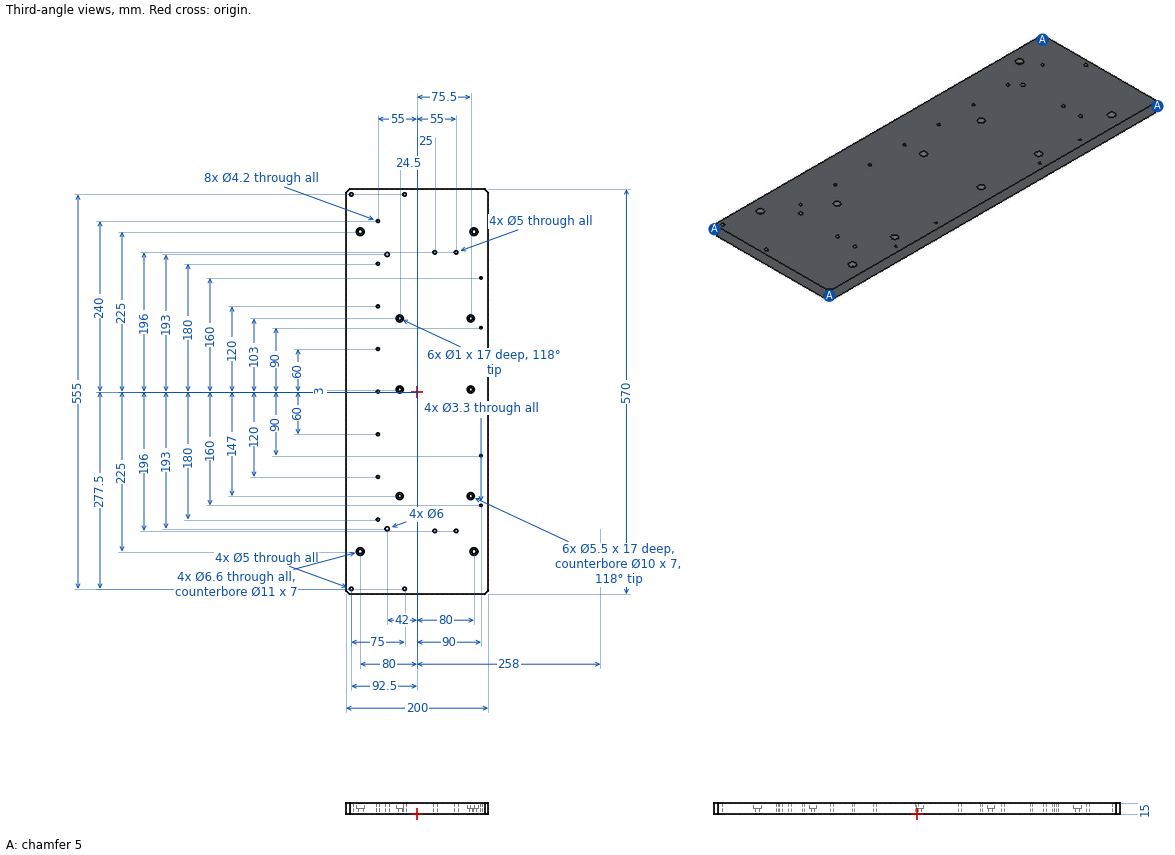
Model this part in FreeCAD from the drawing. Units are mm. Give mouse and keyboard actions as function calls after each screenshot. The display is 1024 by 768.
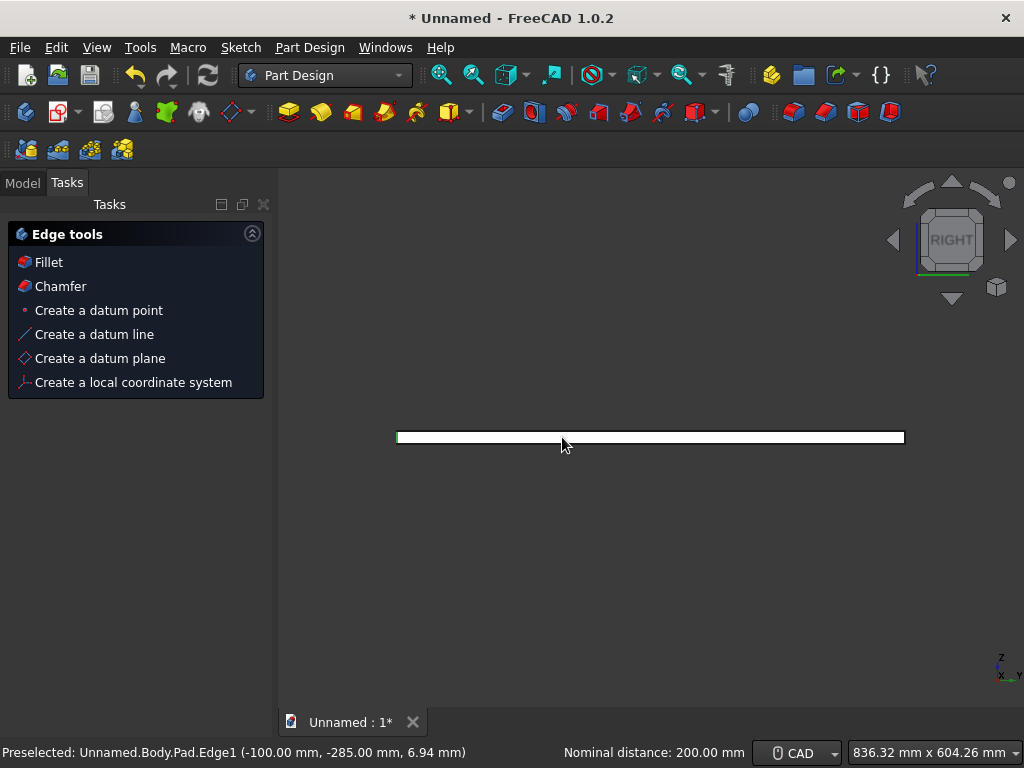
click(905, 436, ctrl)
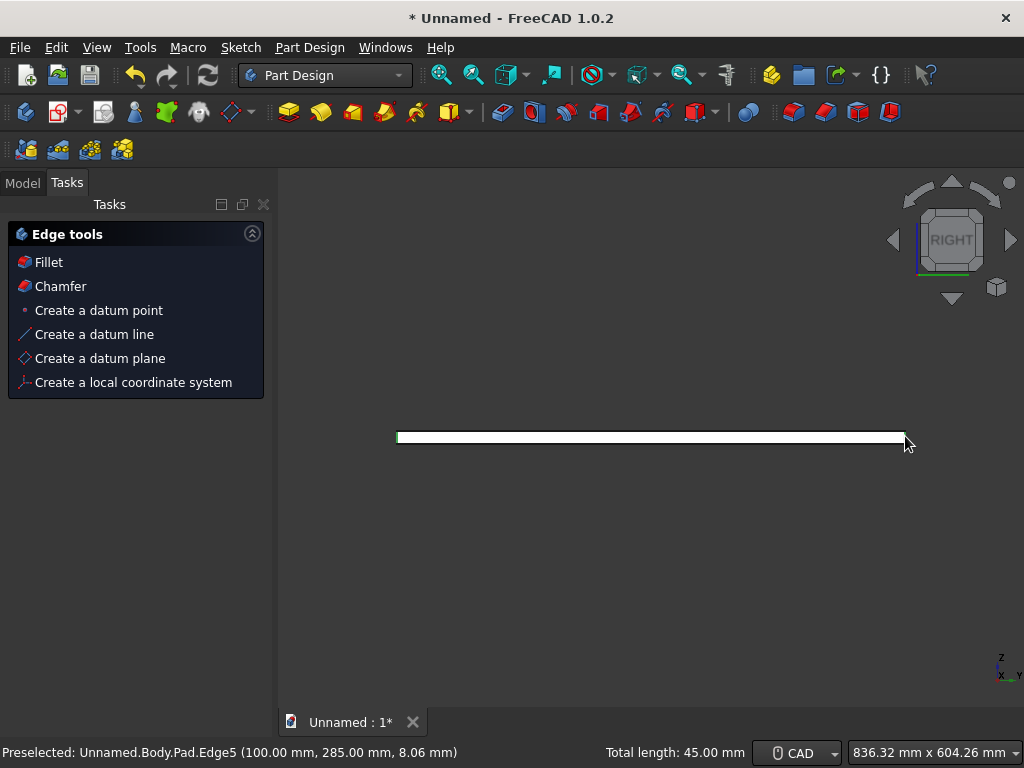
key(5)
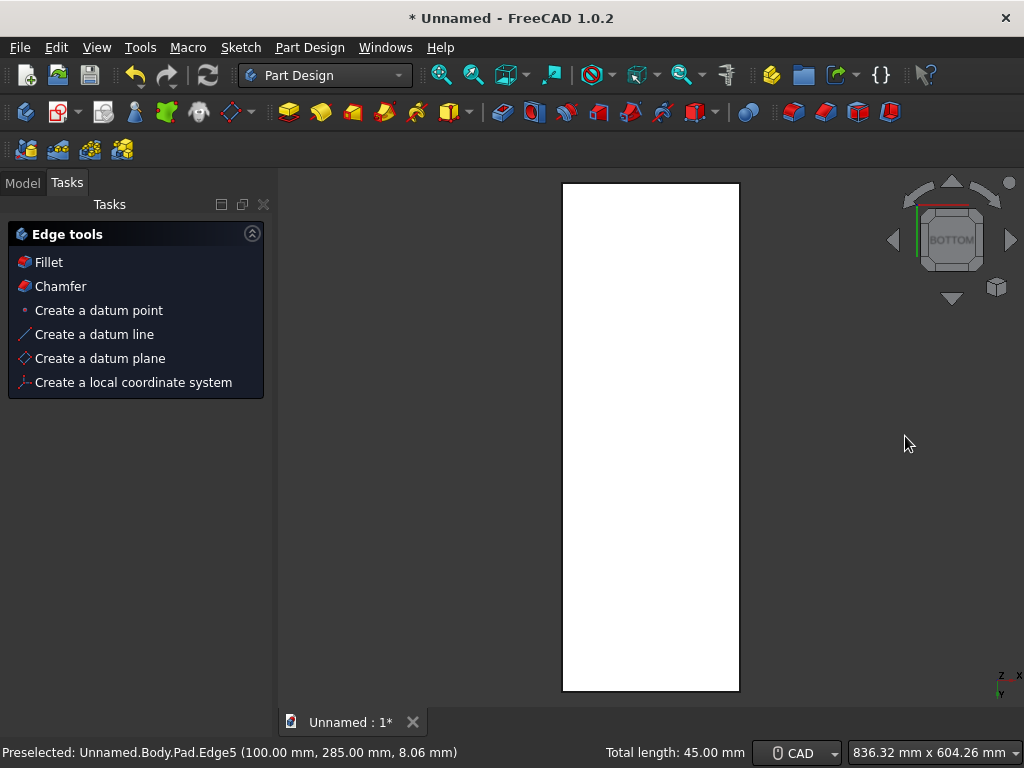
key(4)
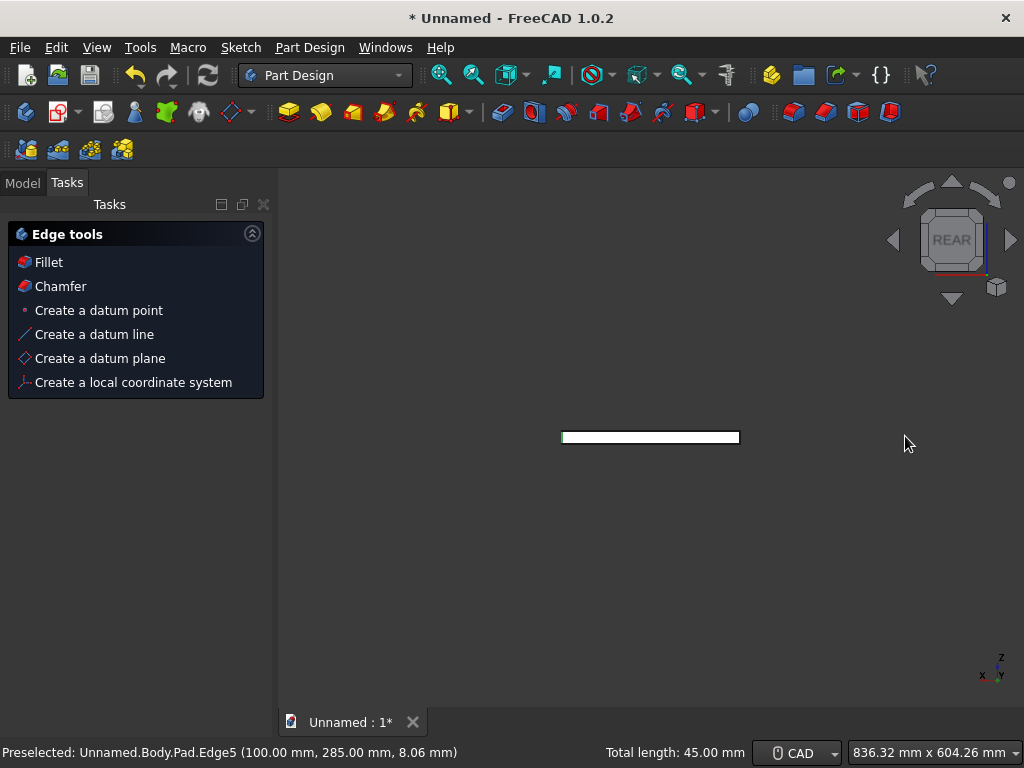
click(442, 76)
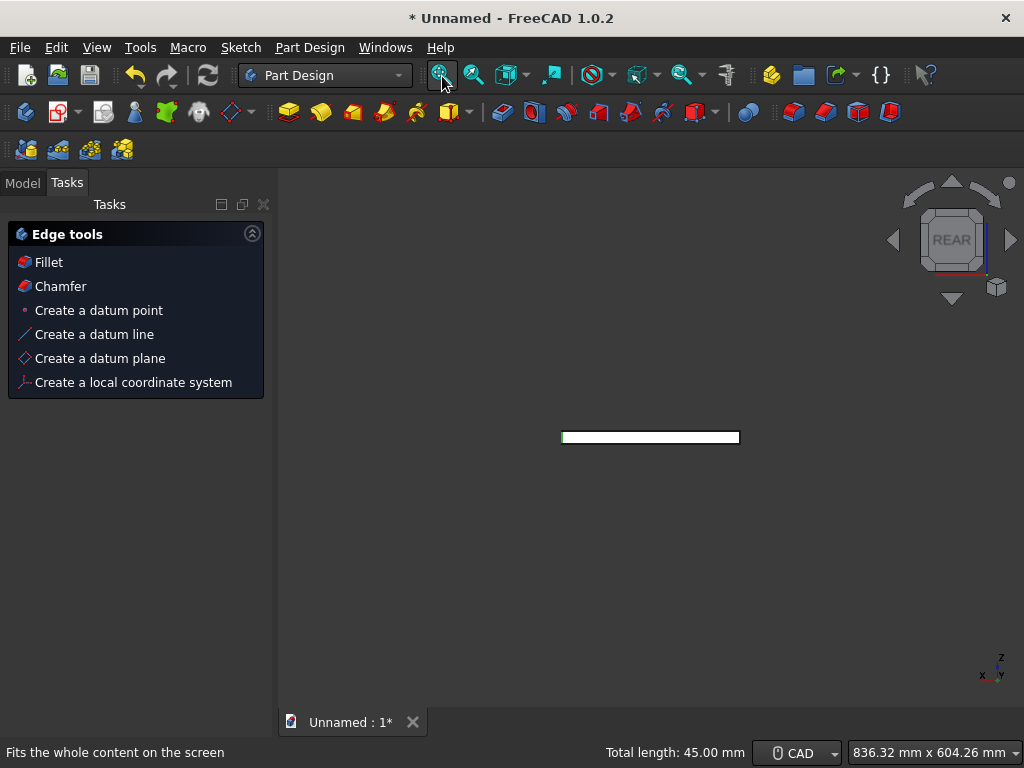
click(740, 437, ctrl)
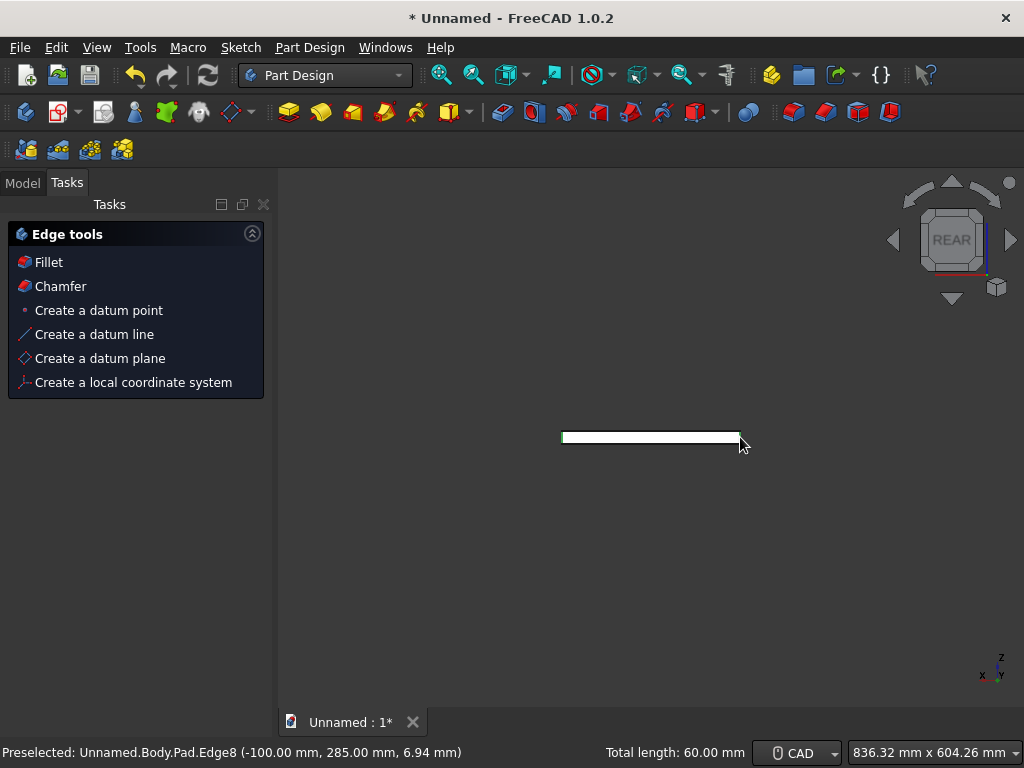
click(826, 112)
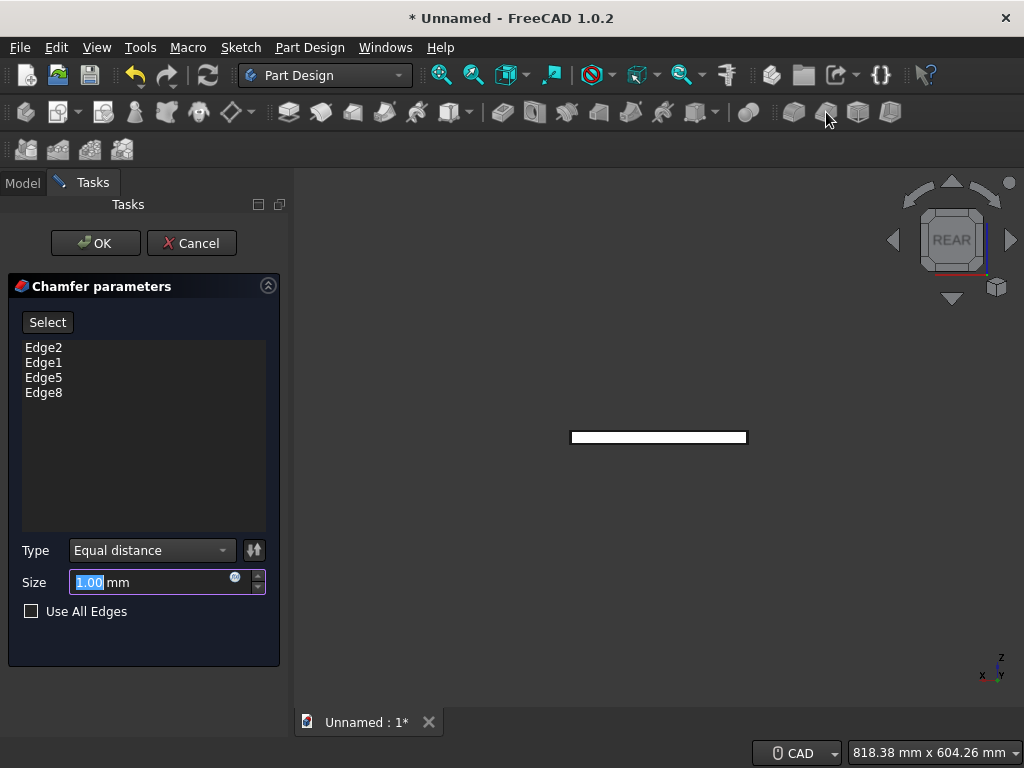
text(5)
key(Tab)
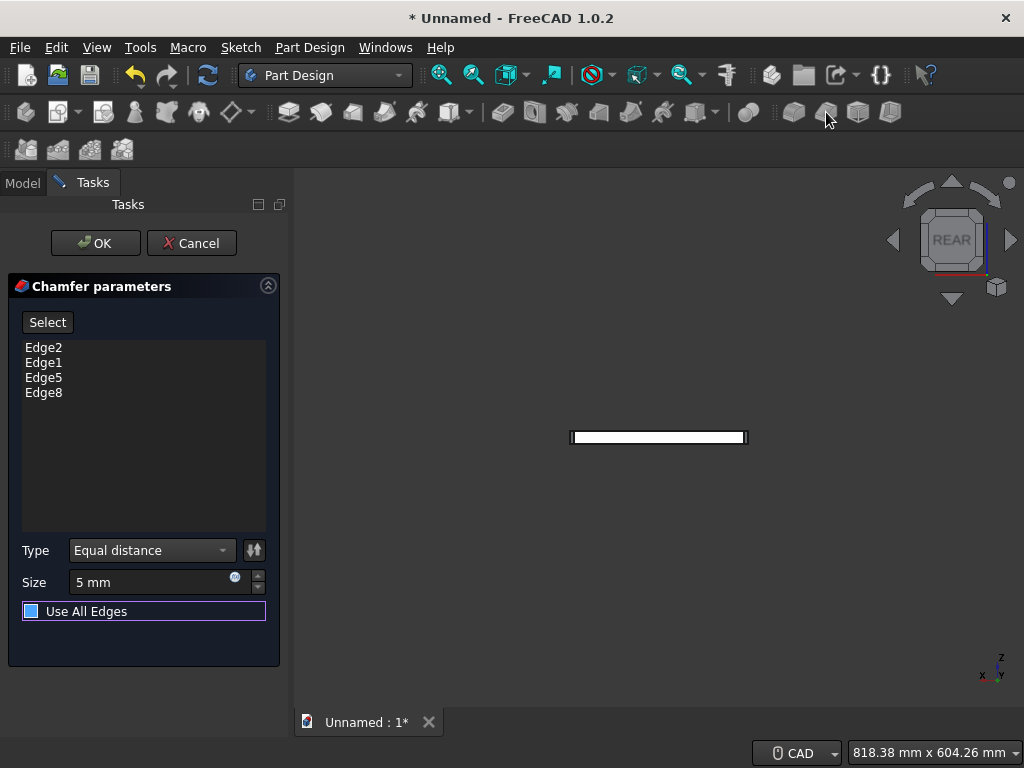
click(96, 243)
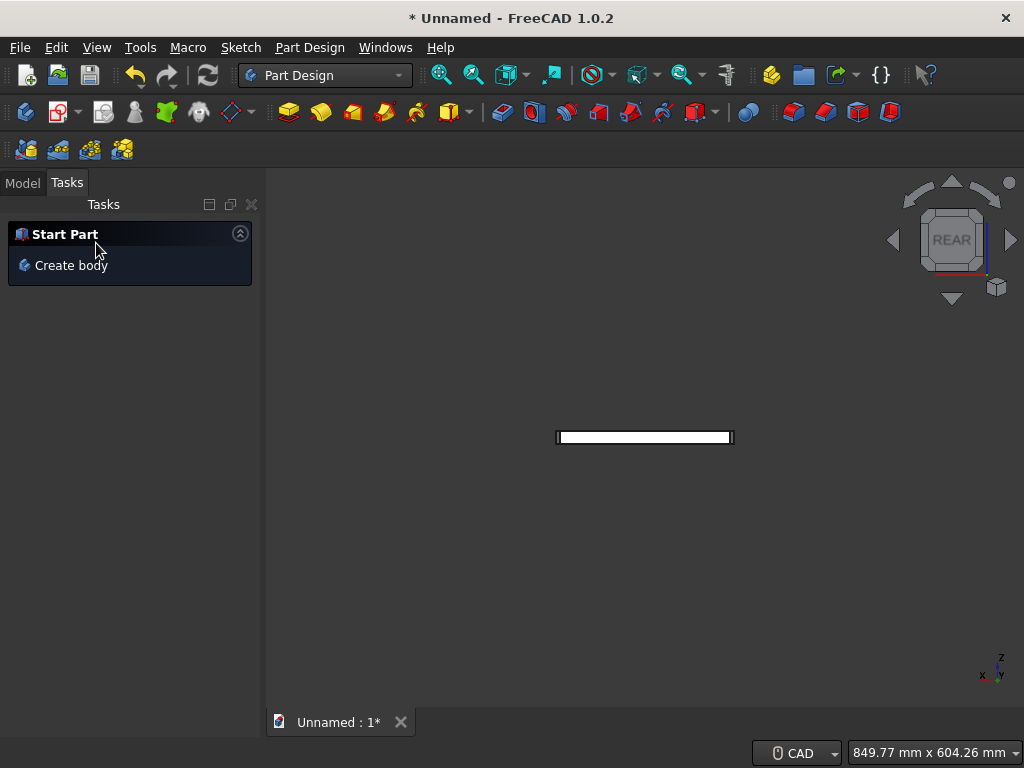
click(442, 76)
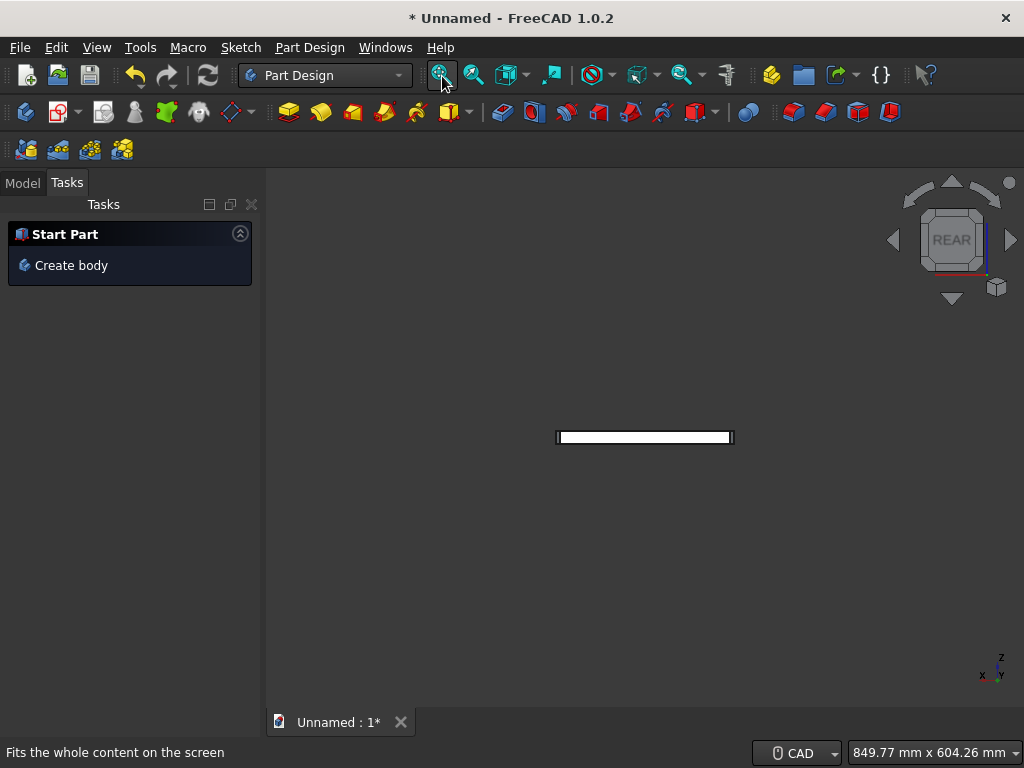
key(0)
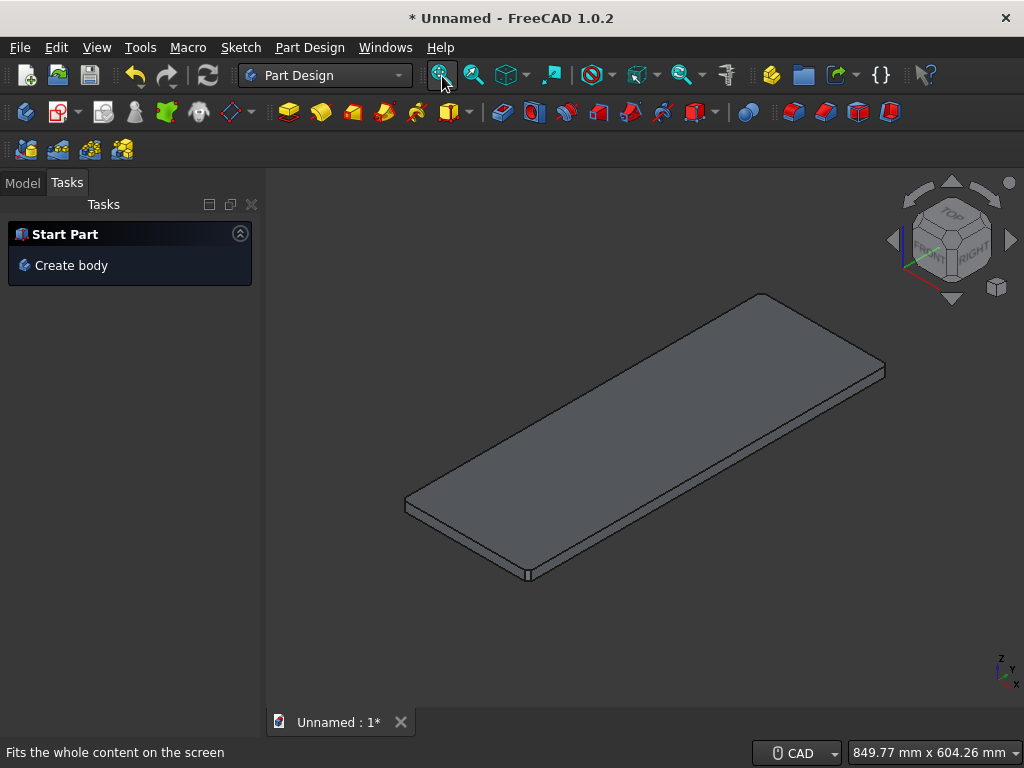
click(748, 372)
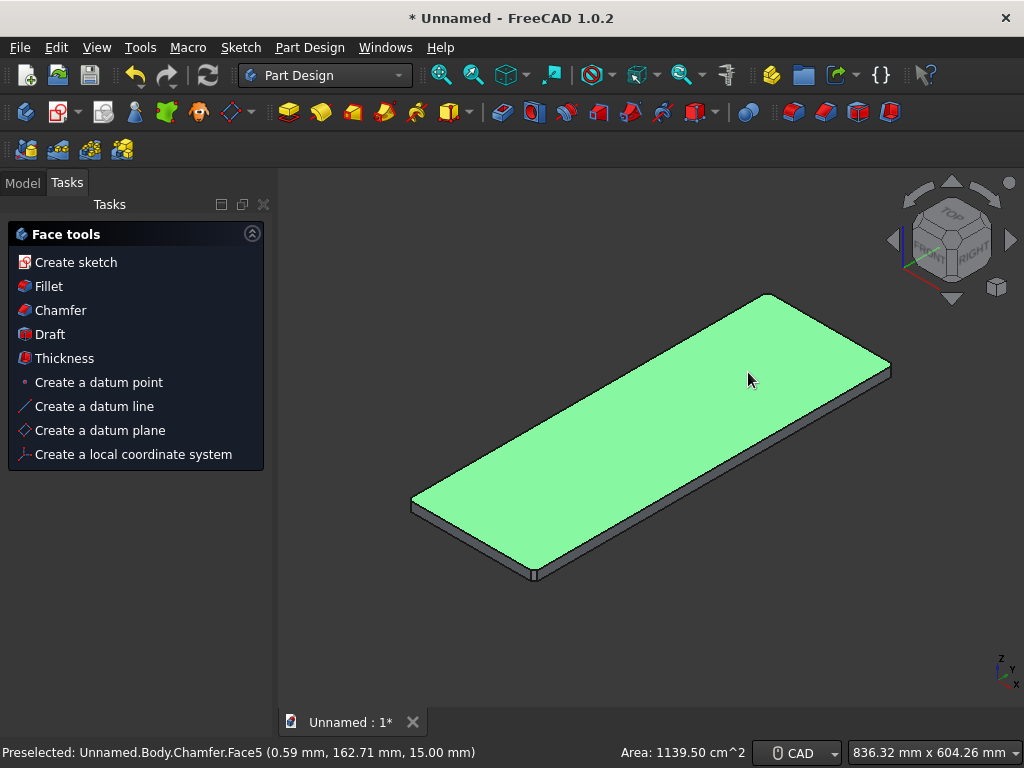
click(58, 112)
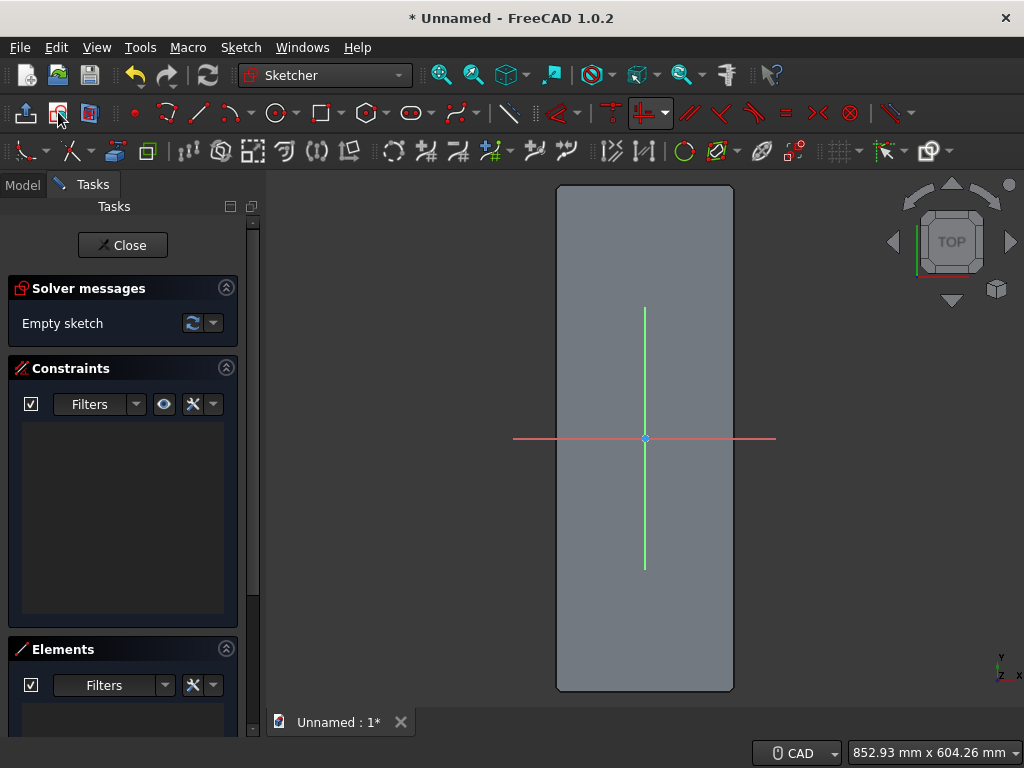
scroll(294, 439, down, 1)